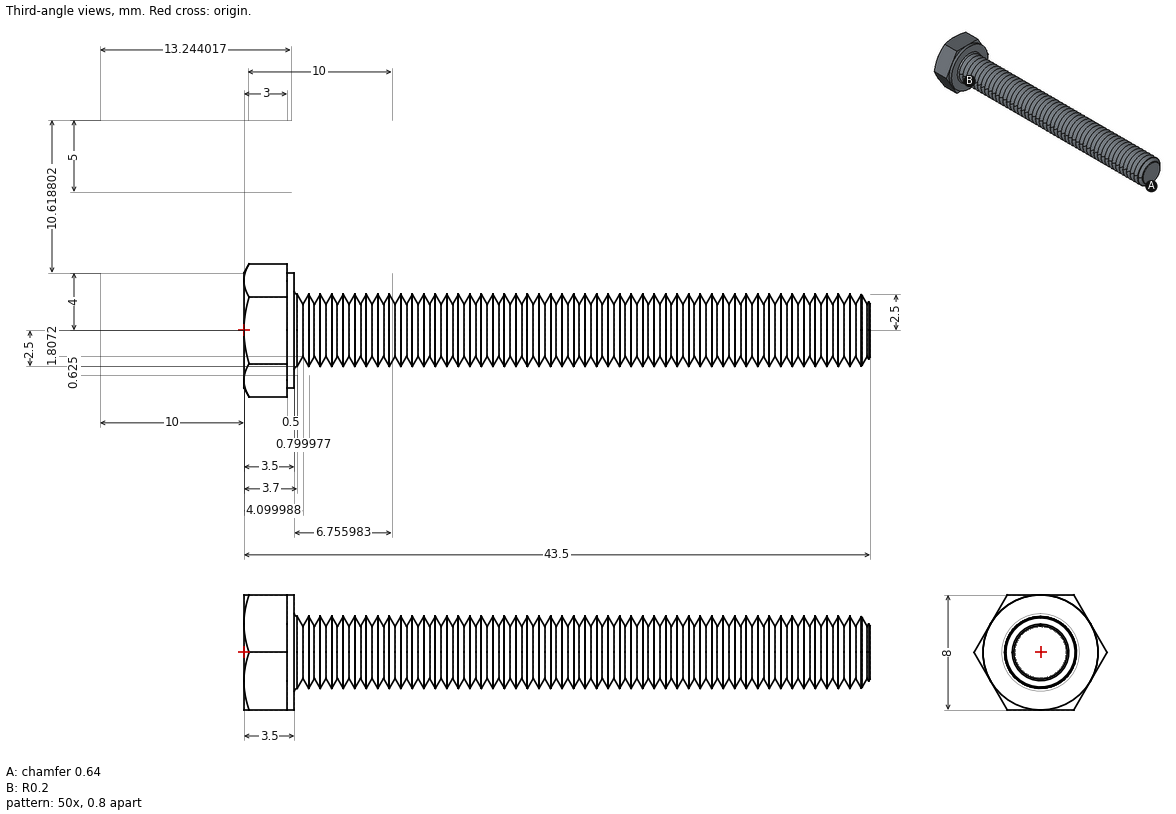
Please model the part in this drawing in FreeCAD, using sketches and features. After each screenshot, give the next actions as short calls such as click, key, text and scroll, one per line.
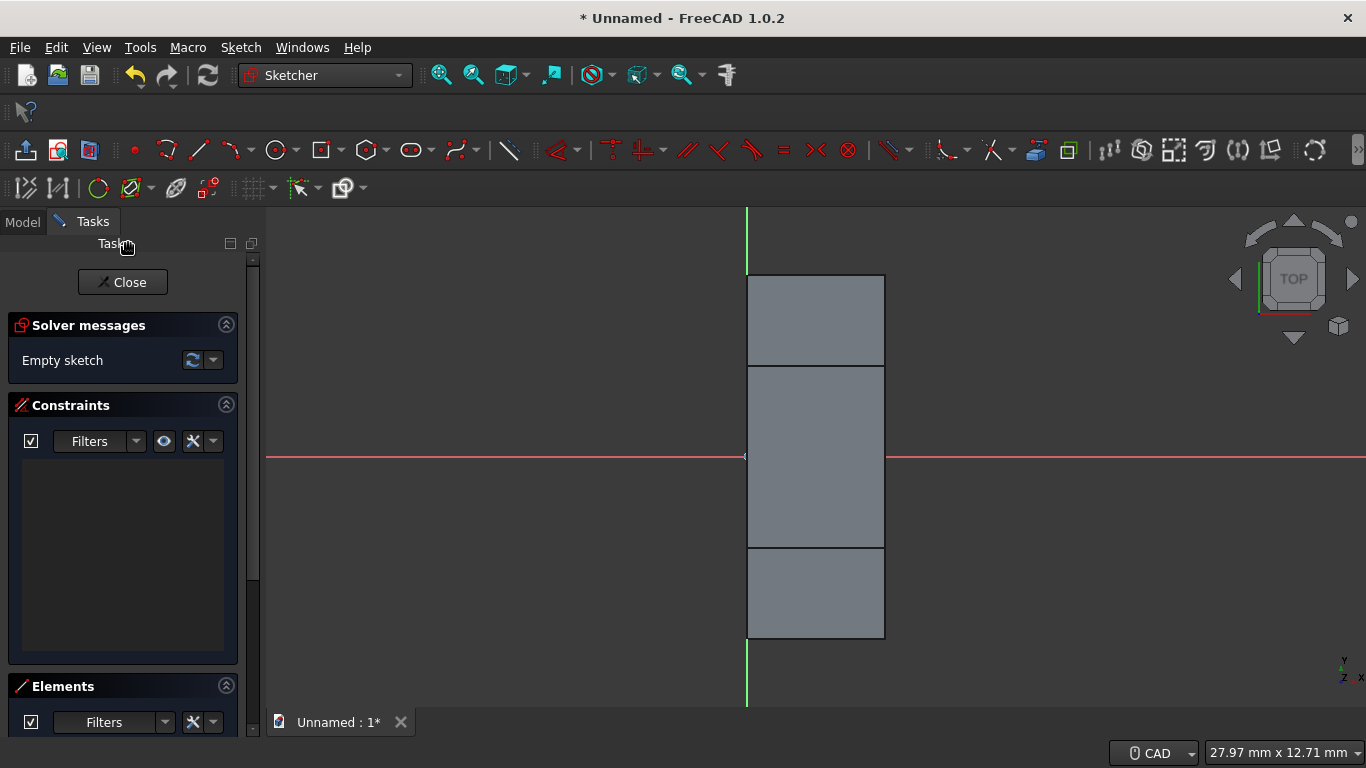
click(90, 150)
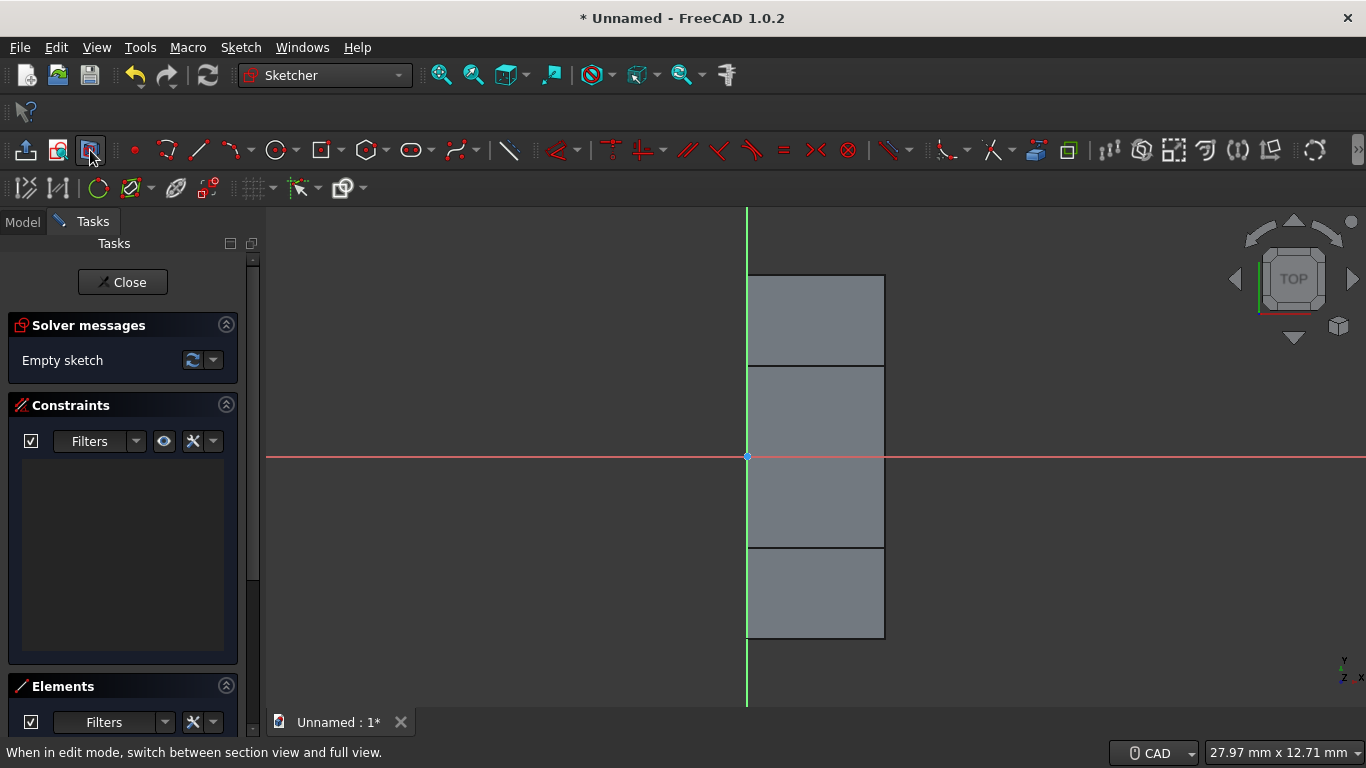
scroll(294, 486, down, 5)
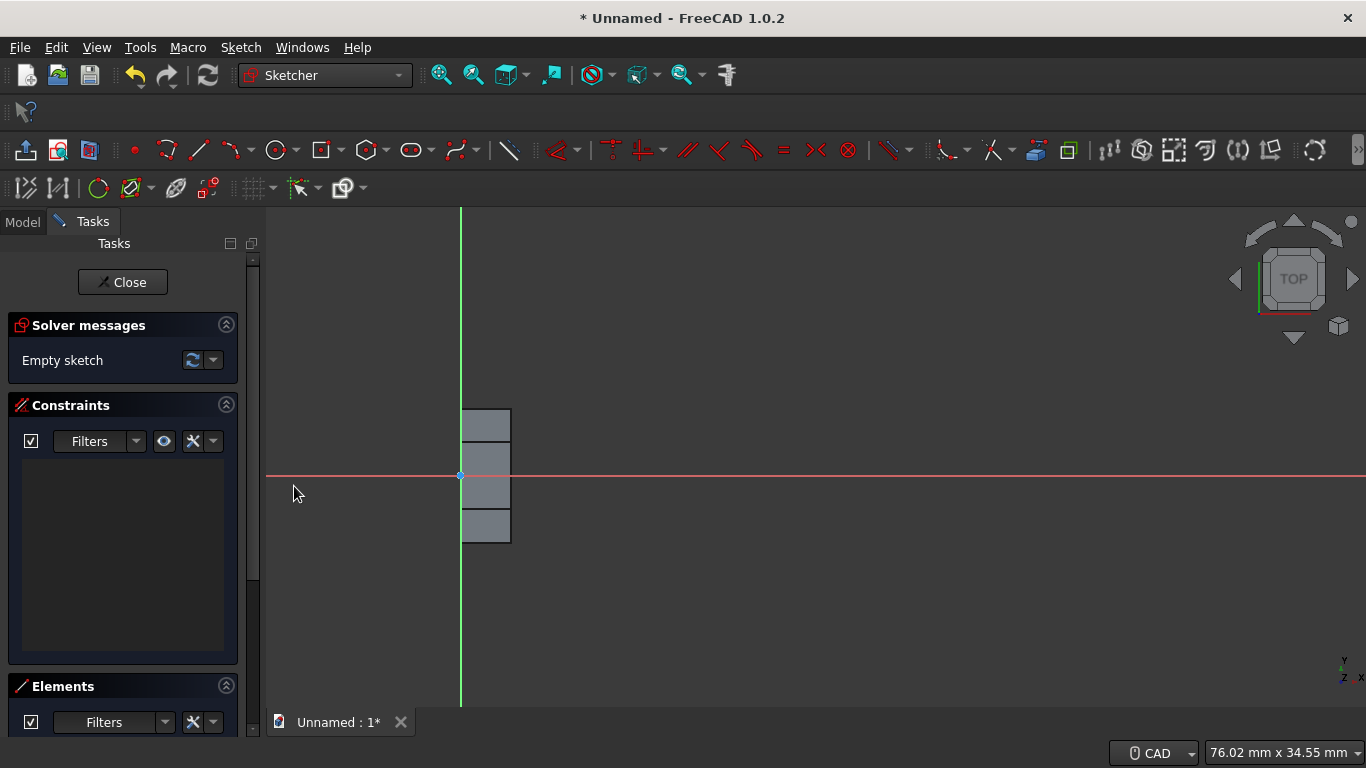
key(g)
key(r)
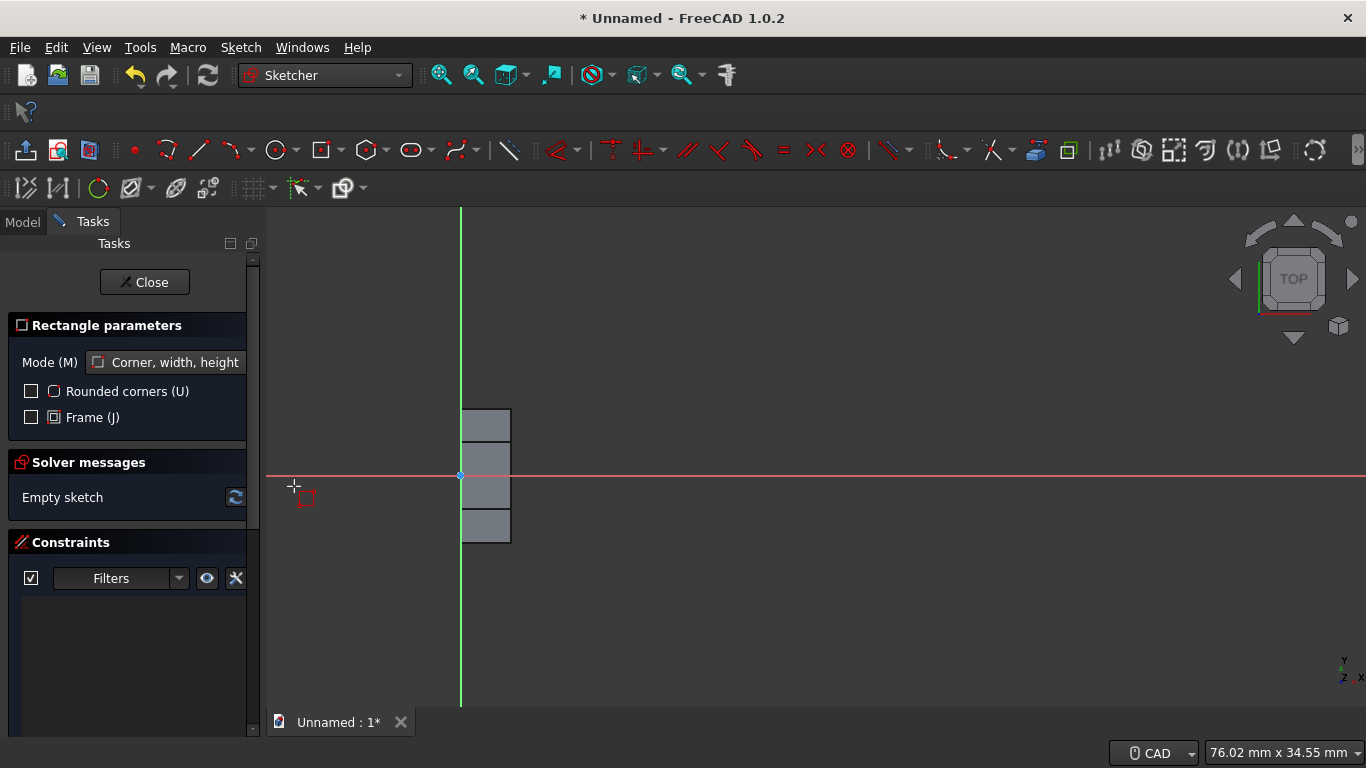
click(461, 476)
move(1090, 440)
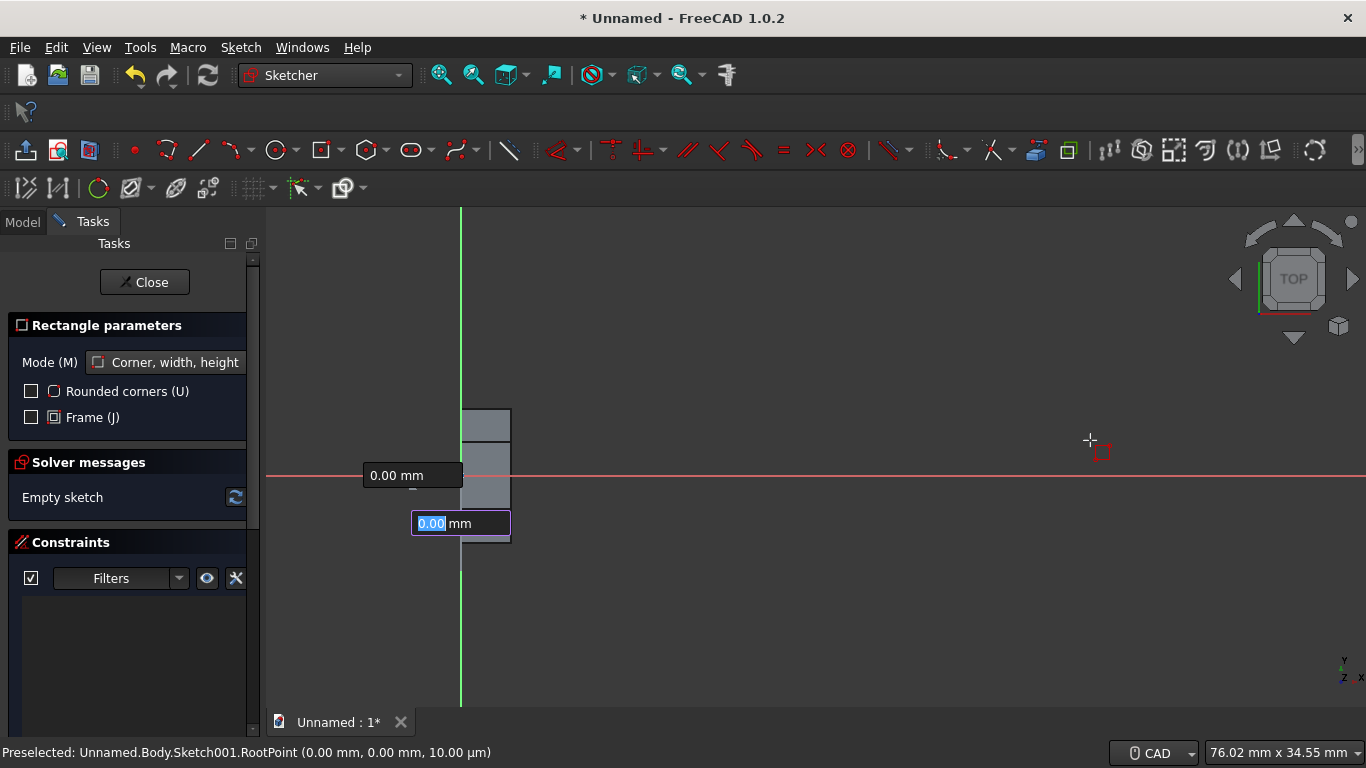
text(43.5)
key(Tab)
text(2.5)
key(Return)
key(Escape)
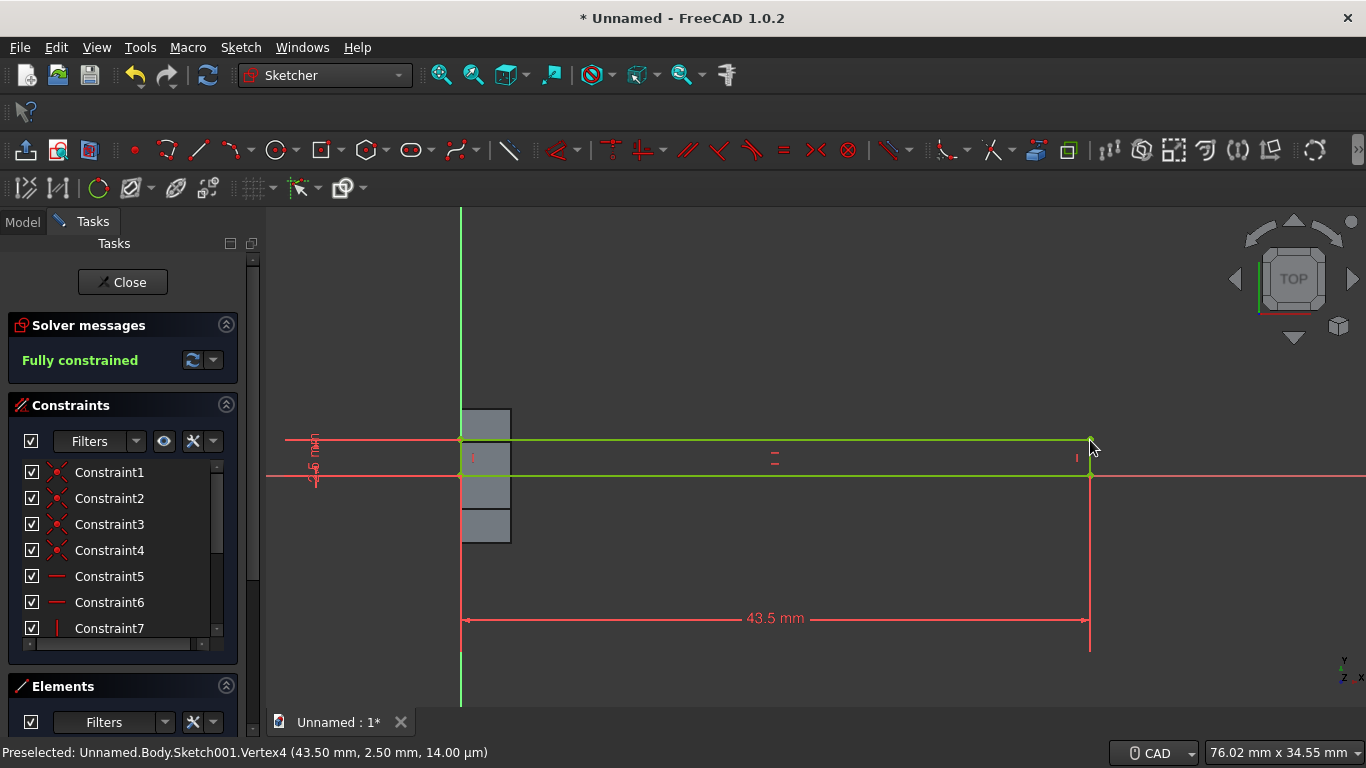
click(123, 282)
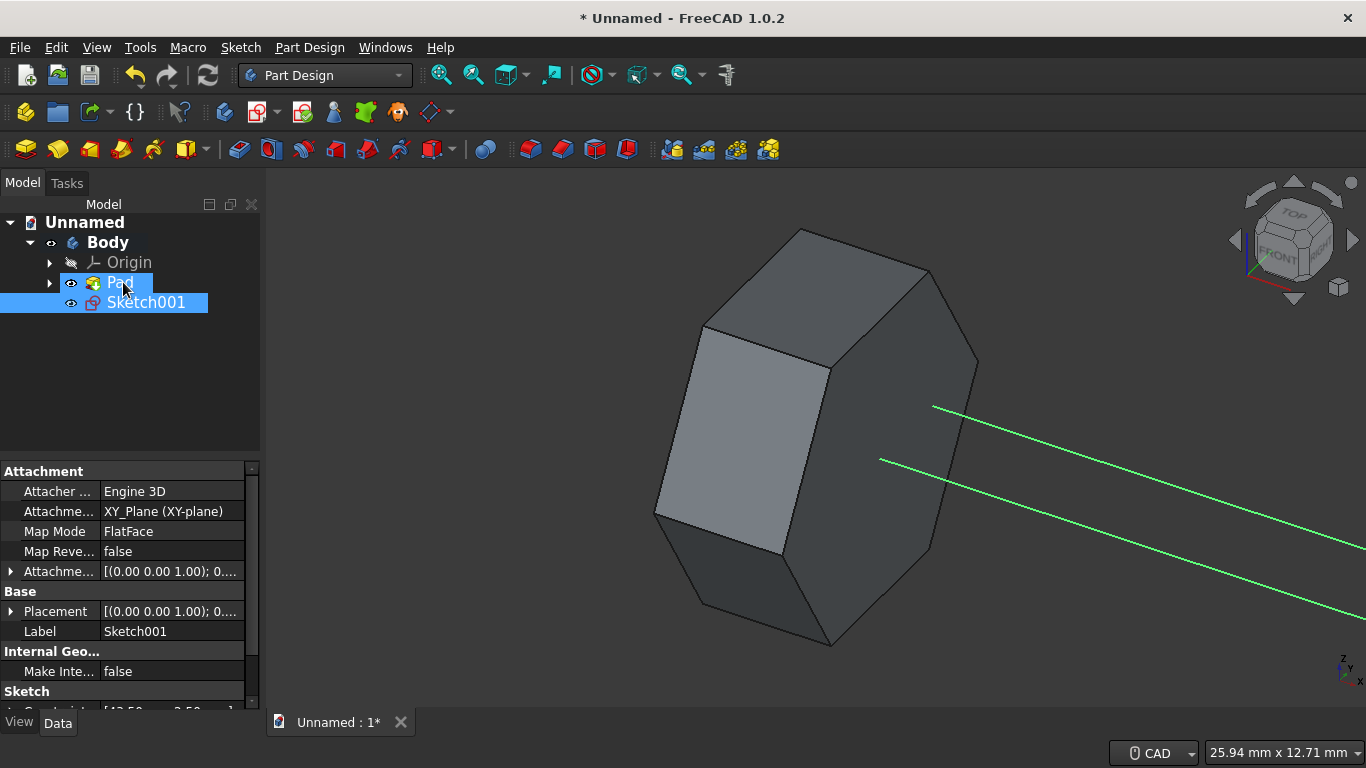
click(58, 150)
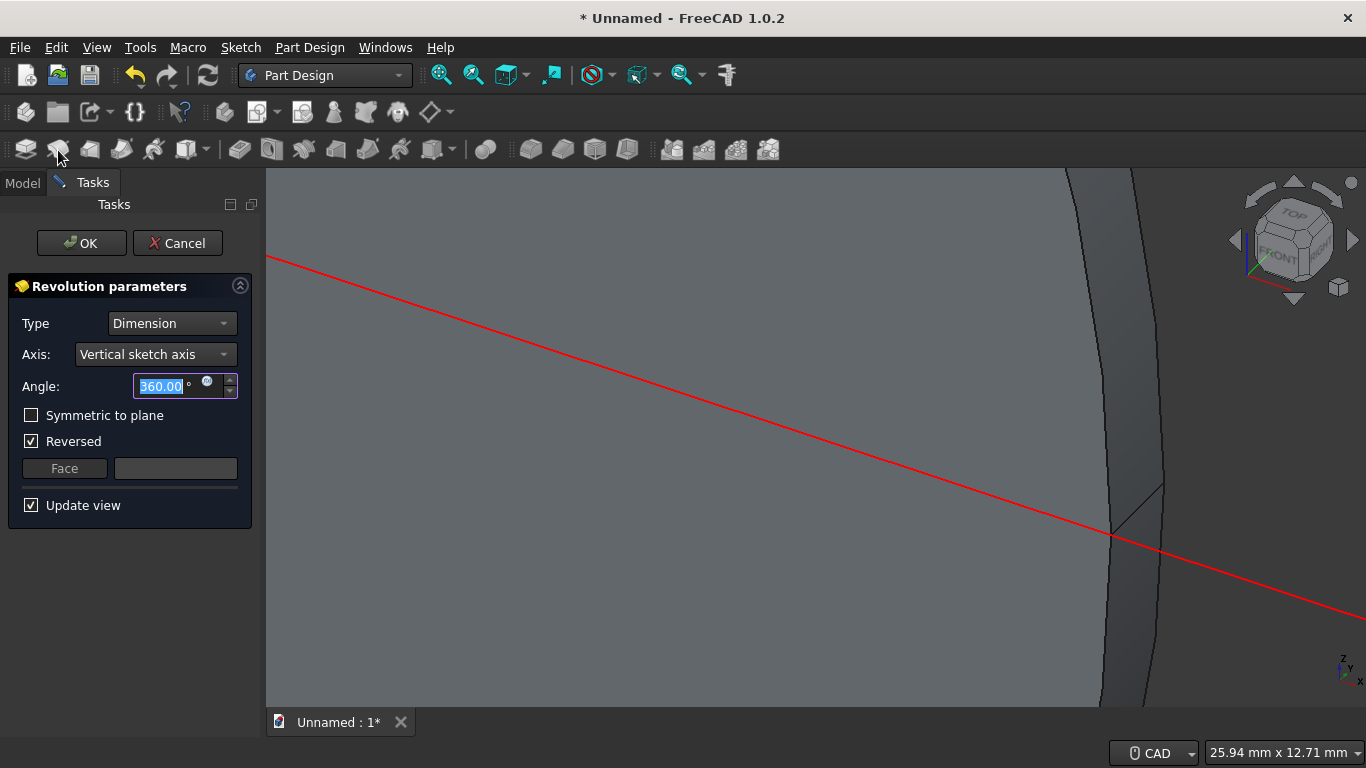
click(156, 354)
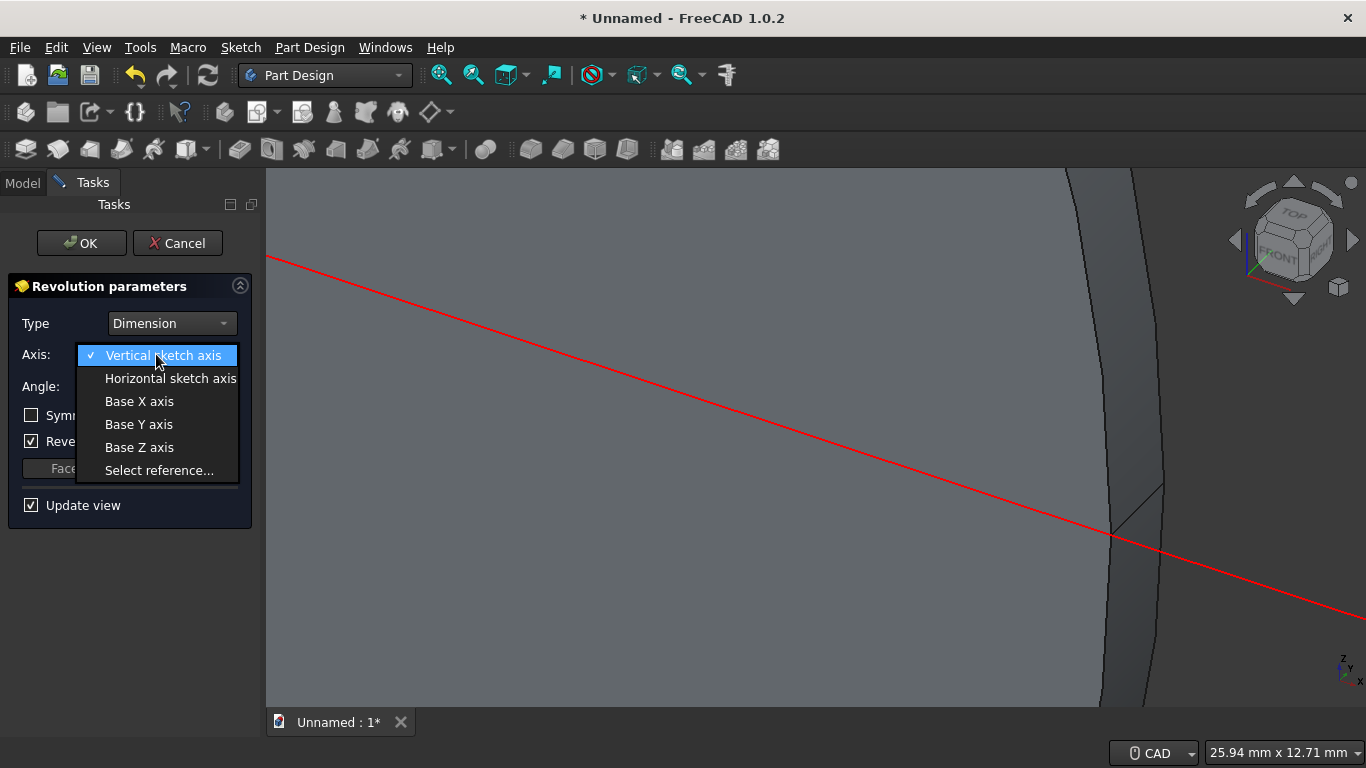
click(156, 378)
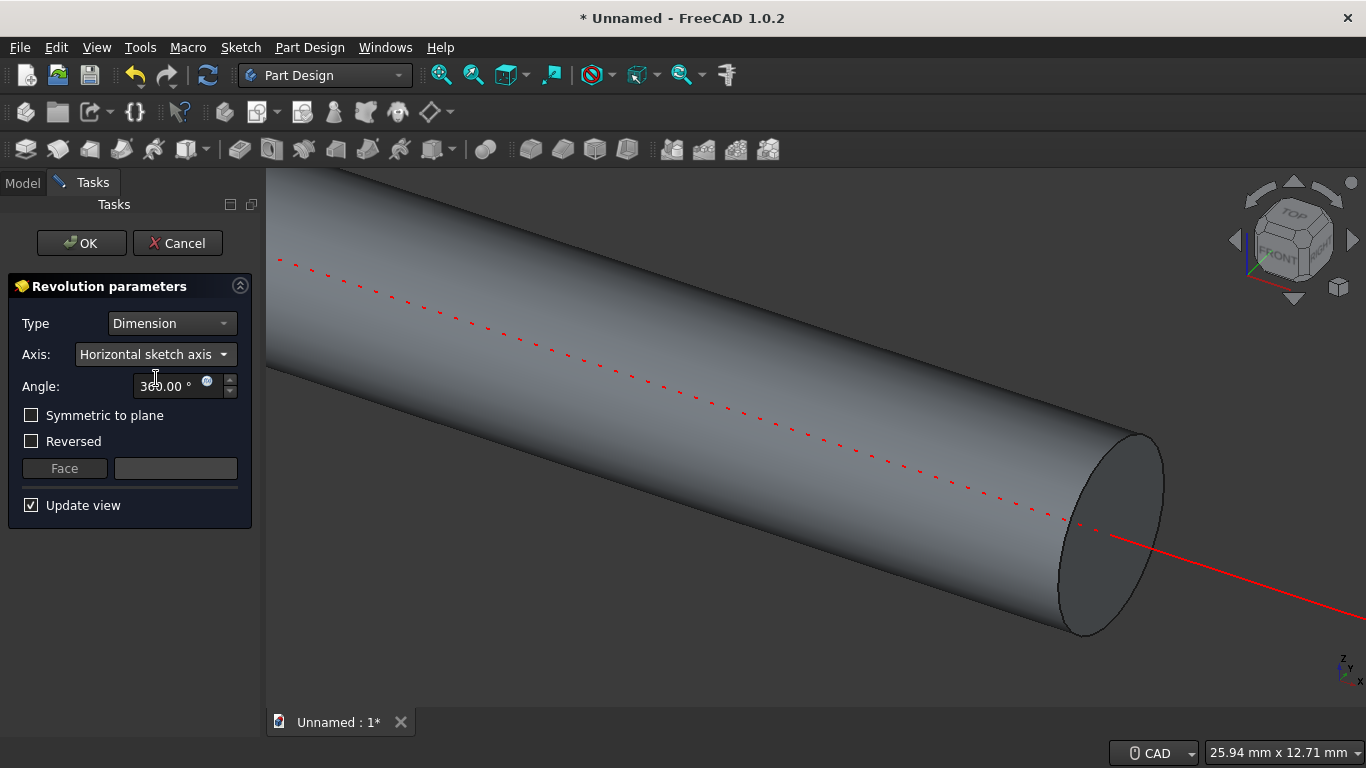
click(82, 243)